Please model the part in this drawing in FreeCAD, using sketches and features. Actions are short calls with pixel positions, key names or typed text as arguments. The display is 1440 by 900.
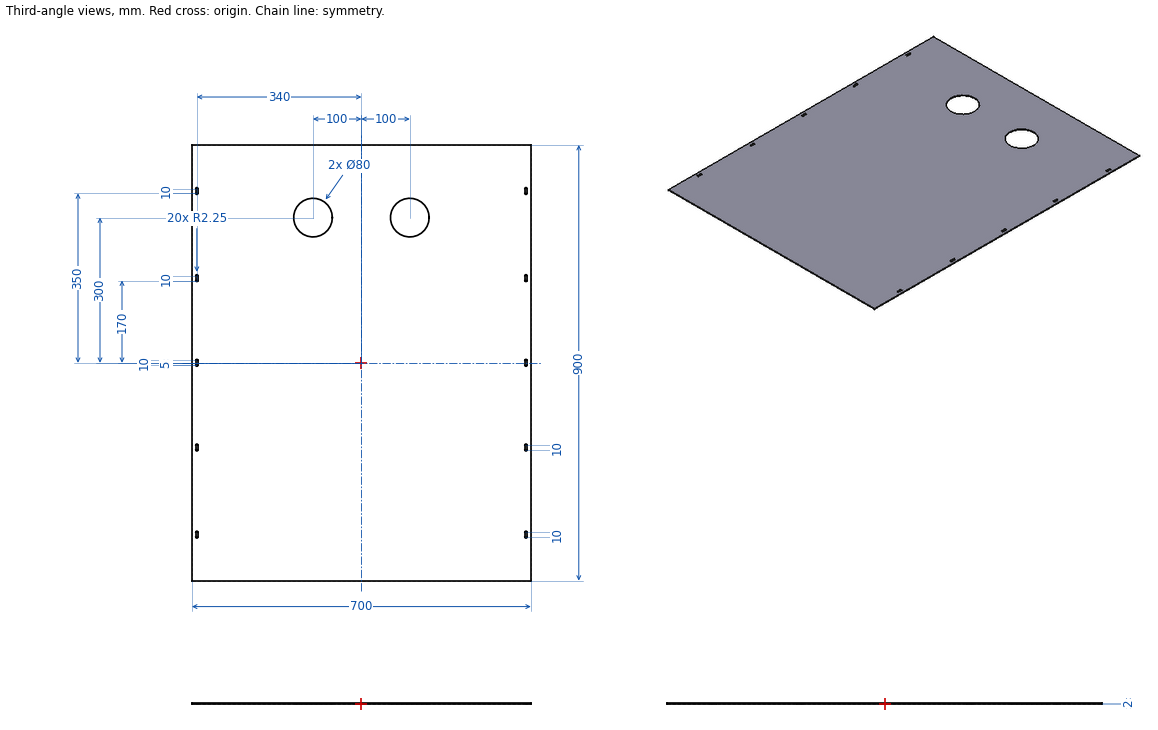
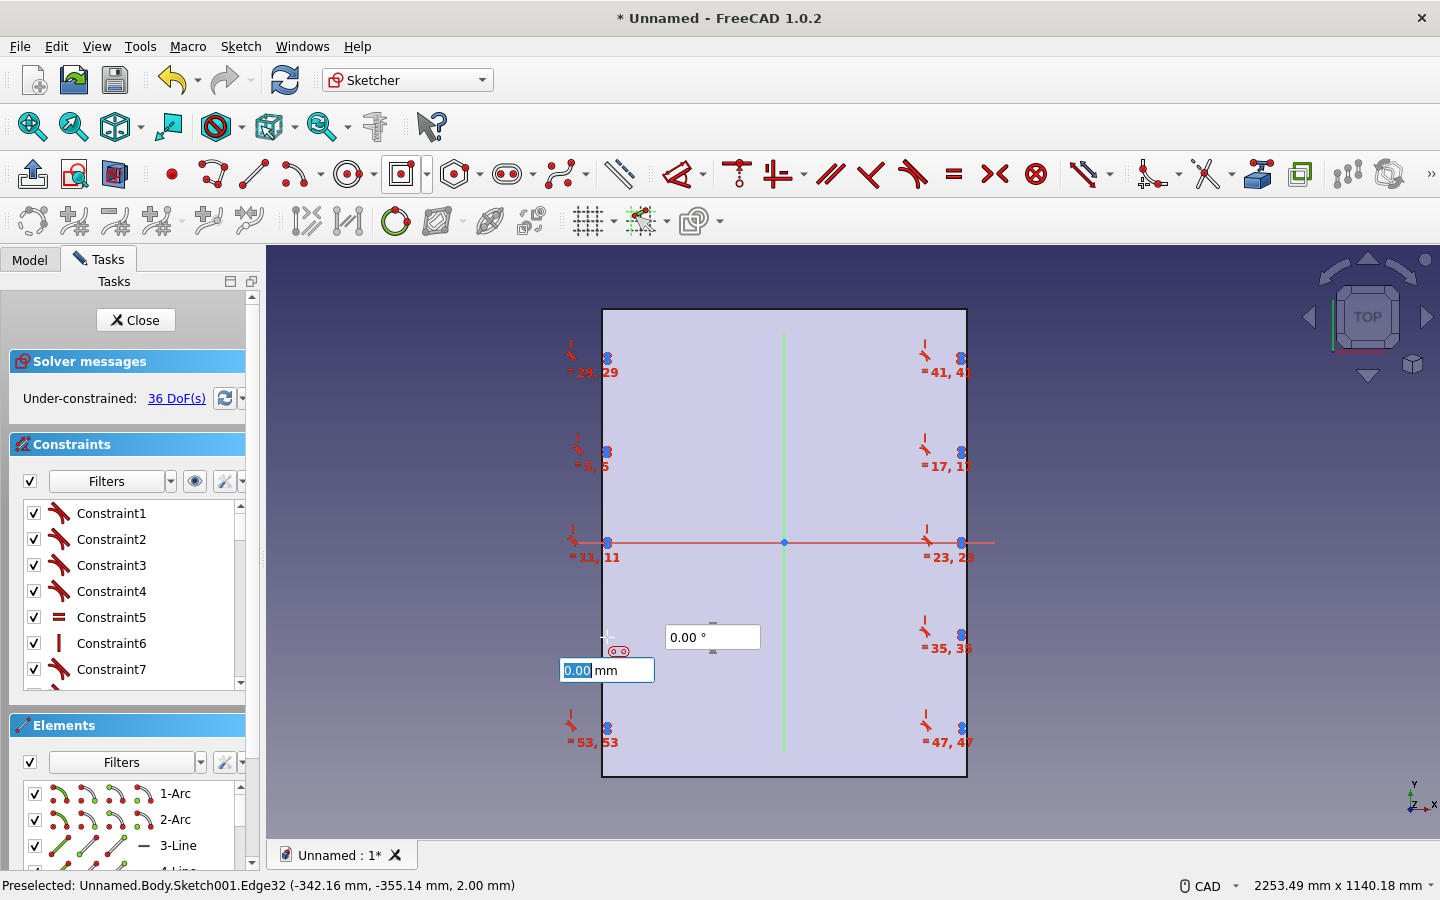
scroll(607, 632, up, 6)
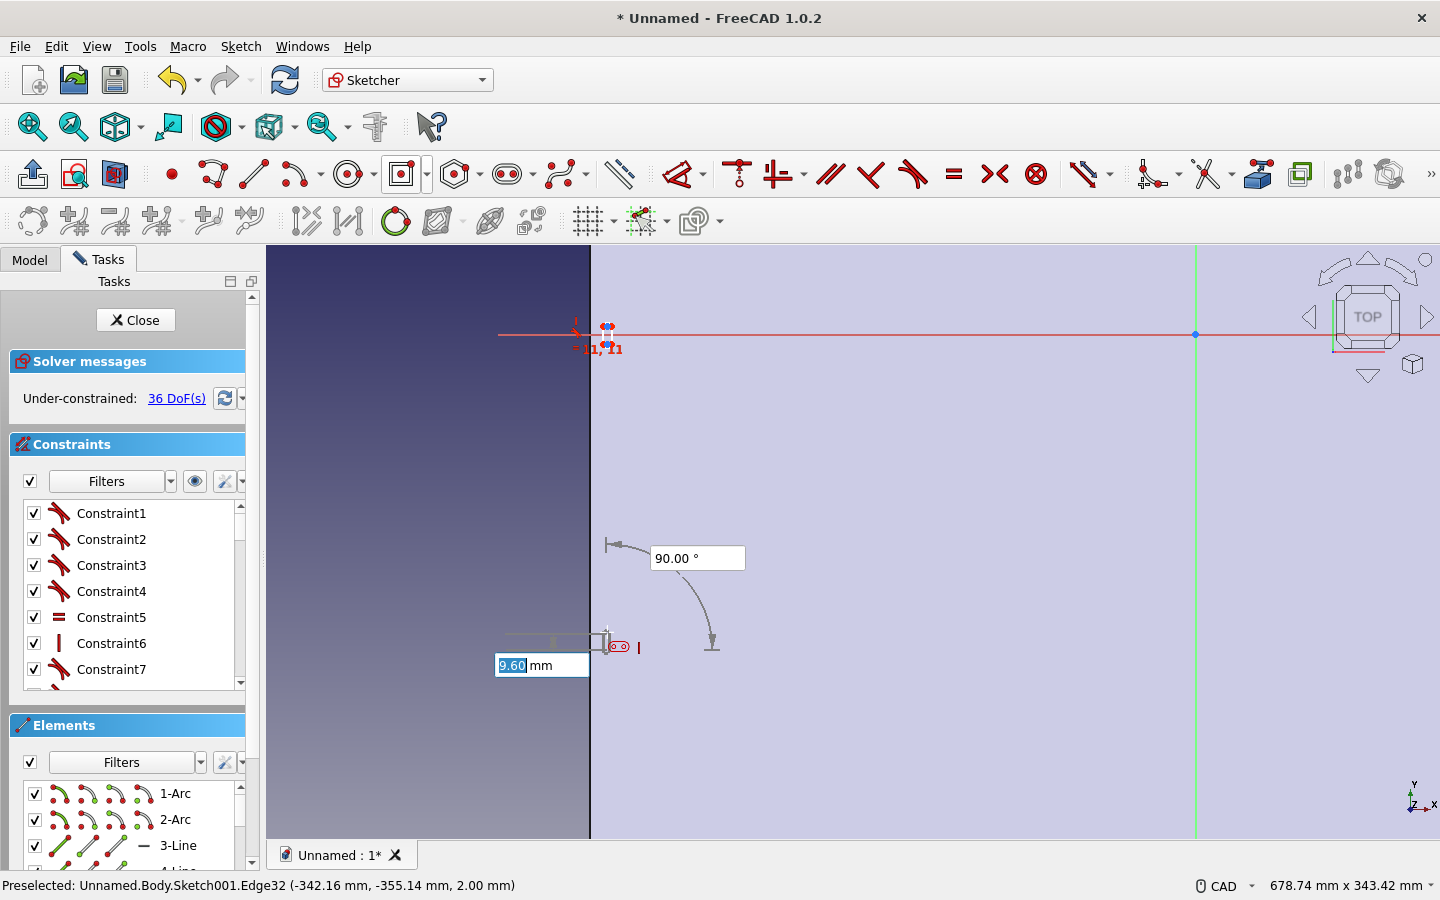
click(606, 629)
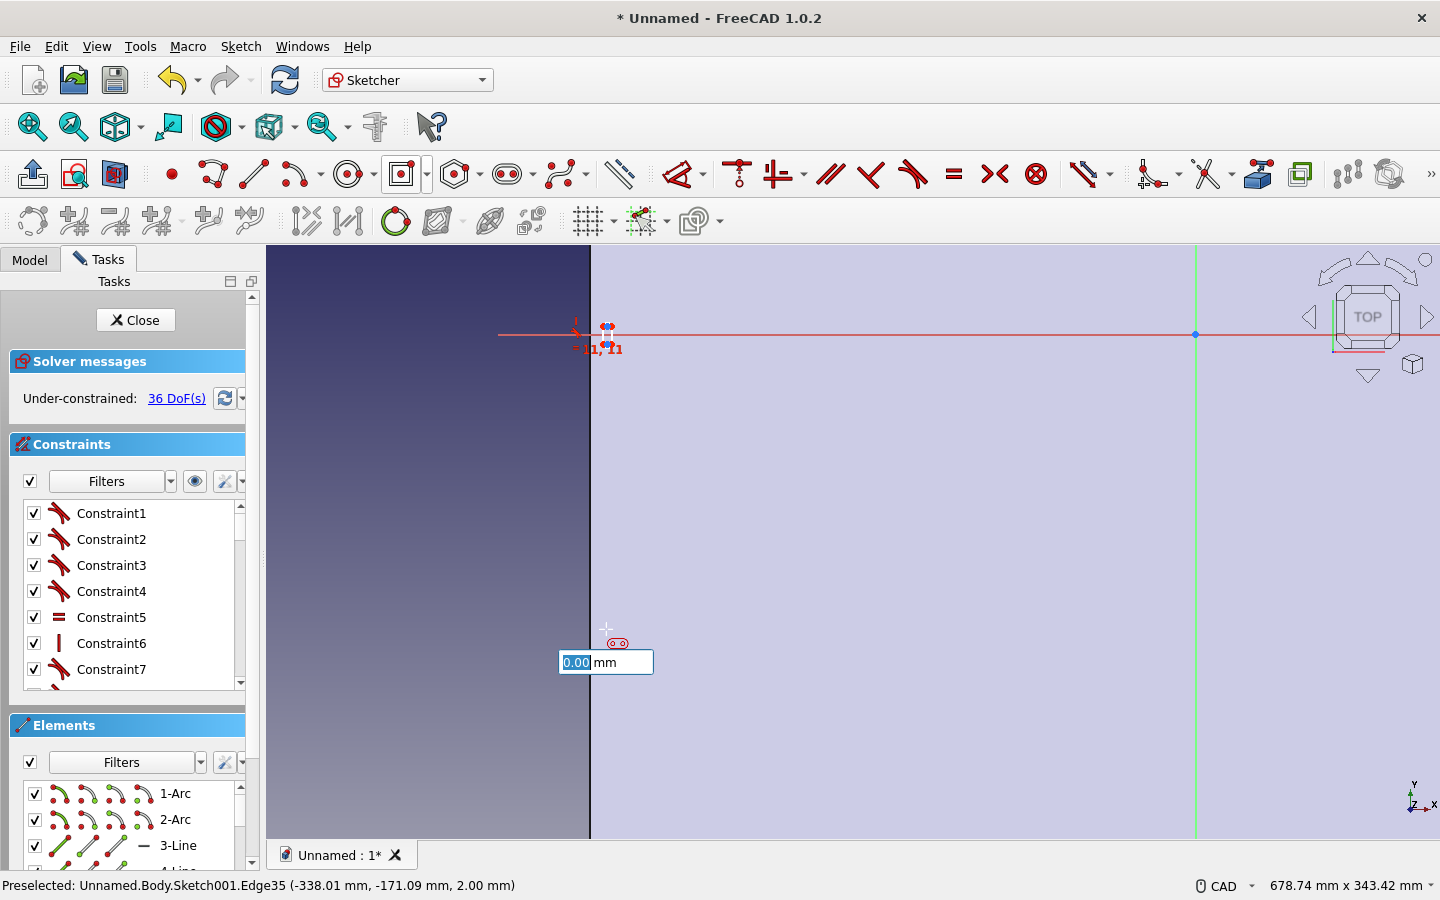
scroll(611, 638, up, 8)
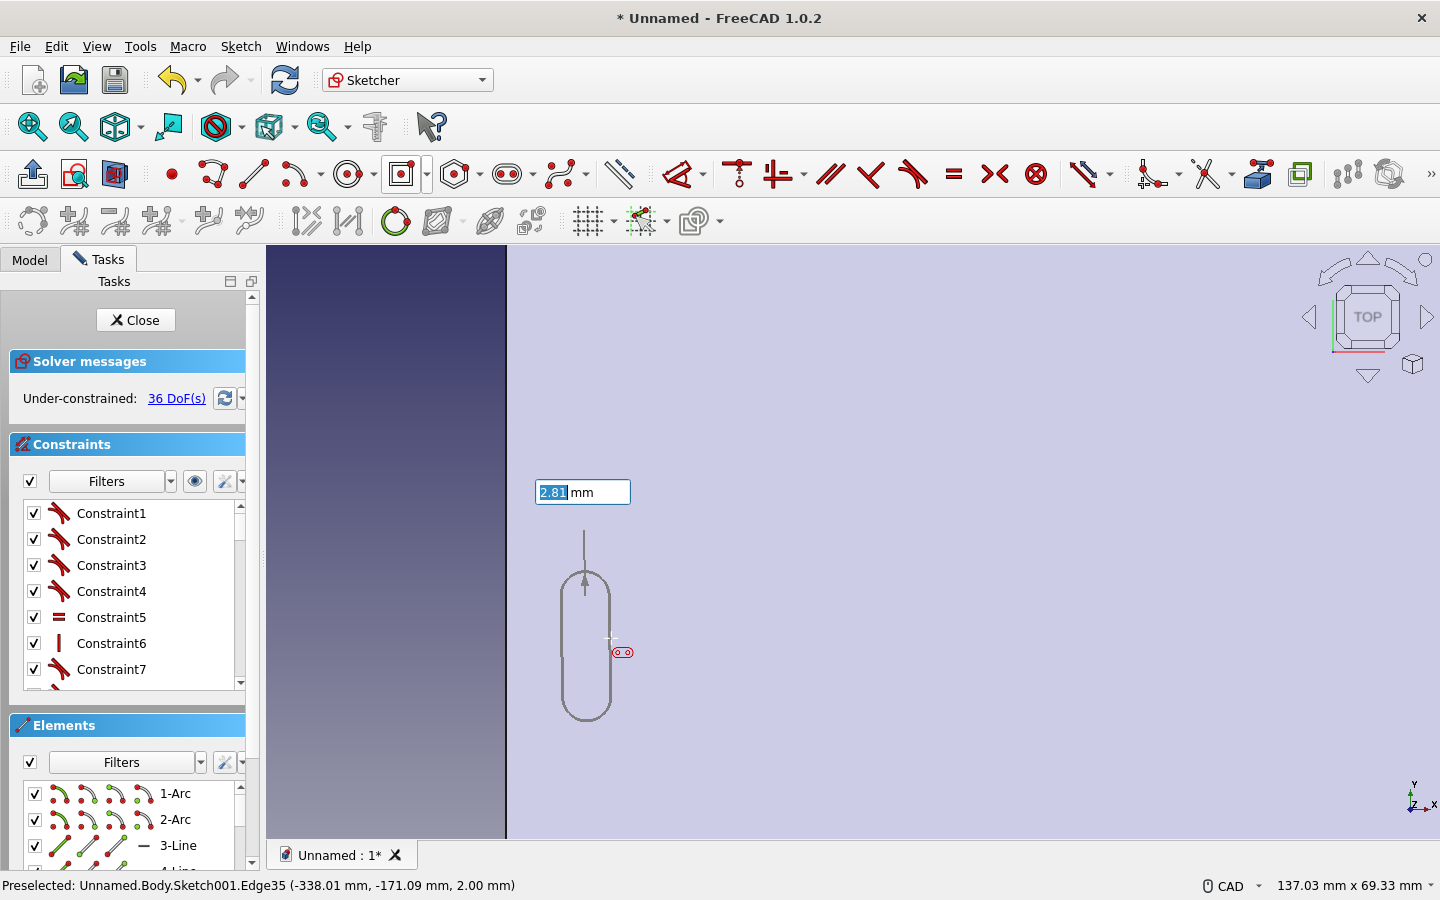
click(611, 634)
key(Escape)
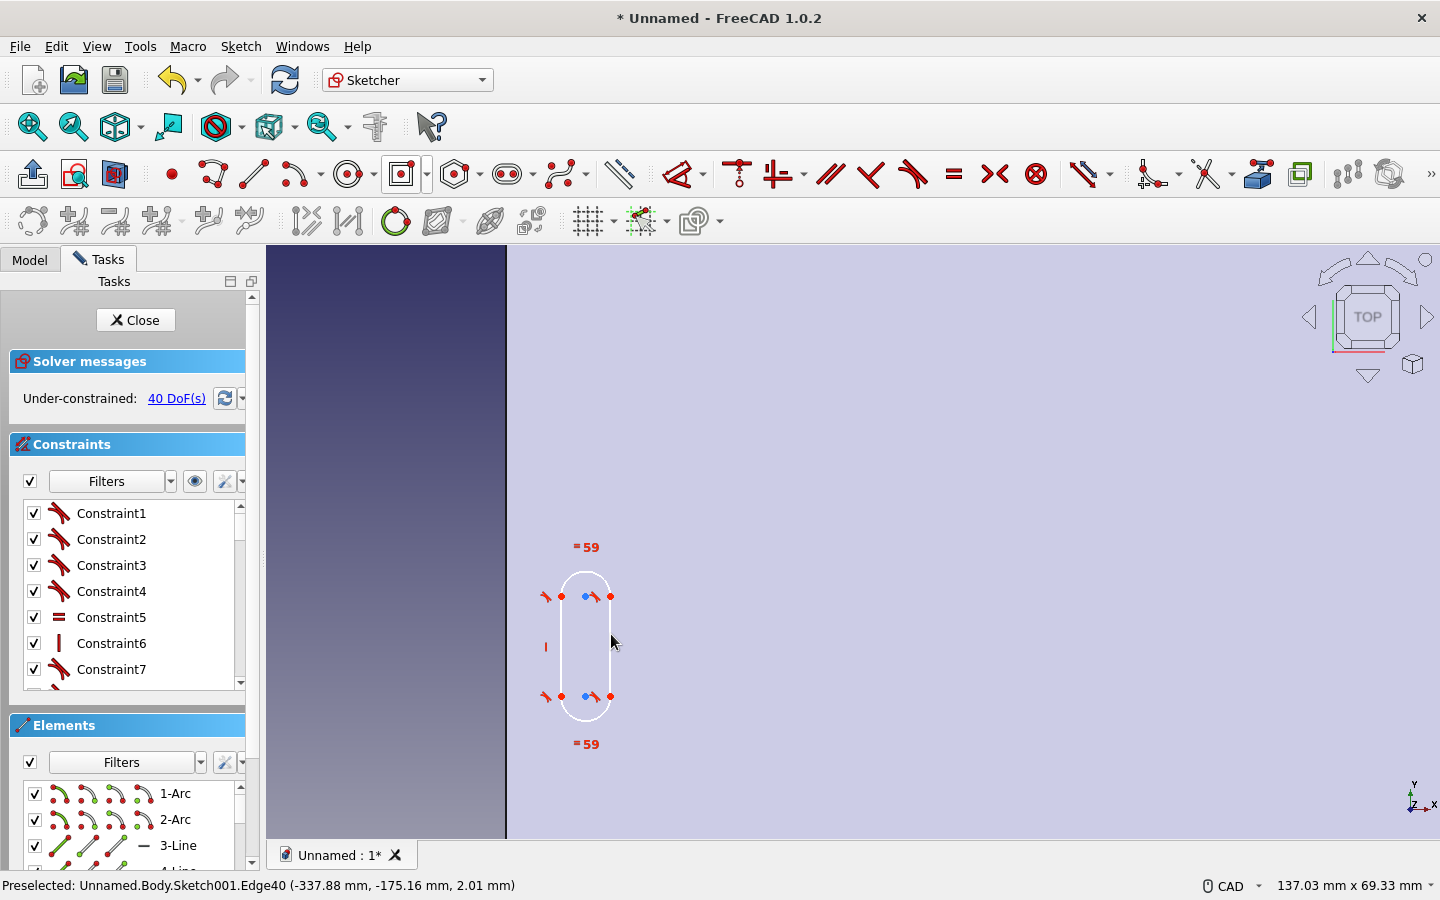
scroll(608, 633, down, 14)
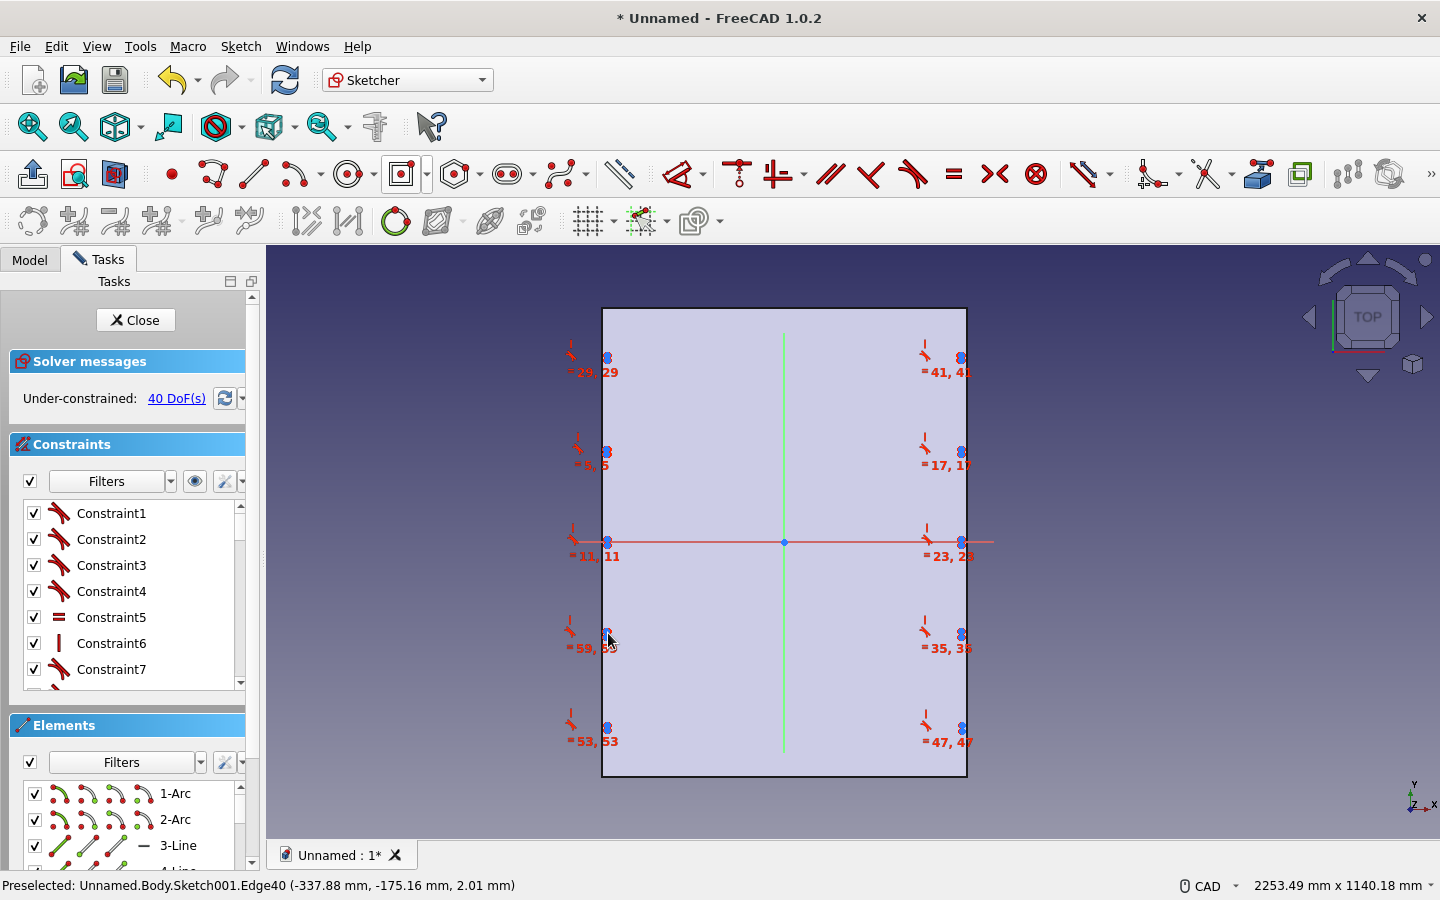
scroll(606, 456, up, 12)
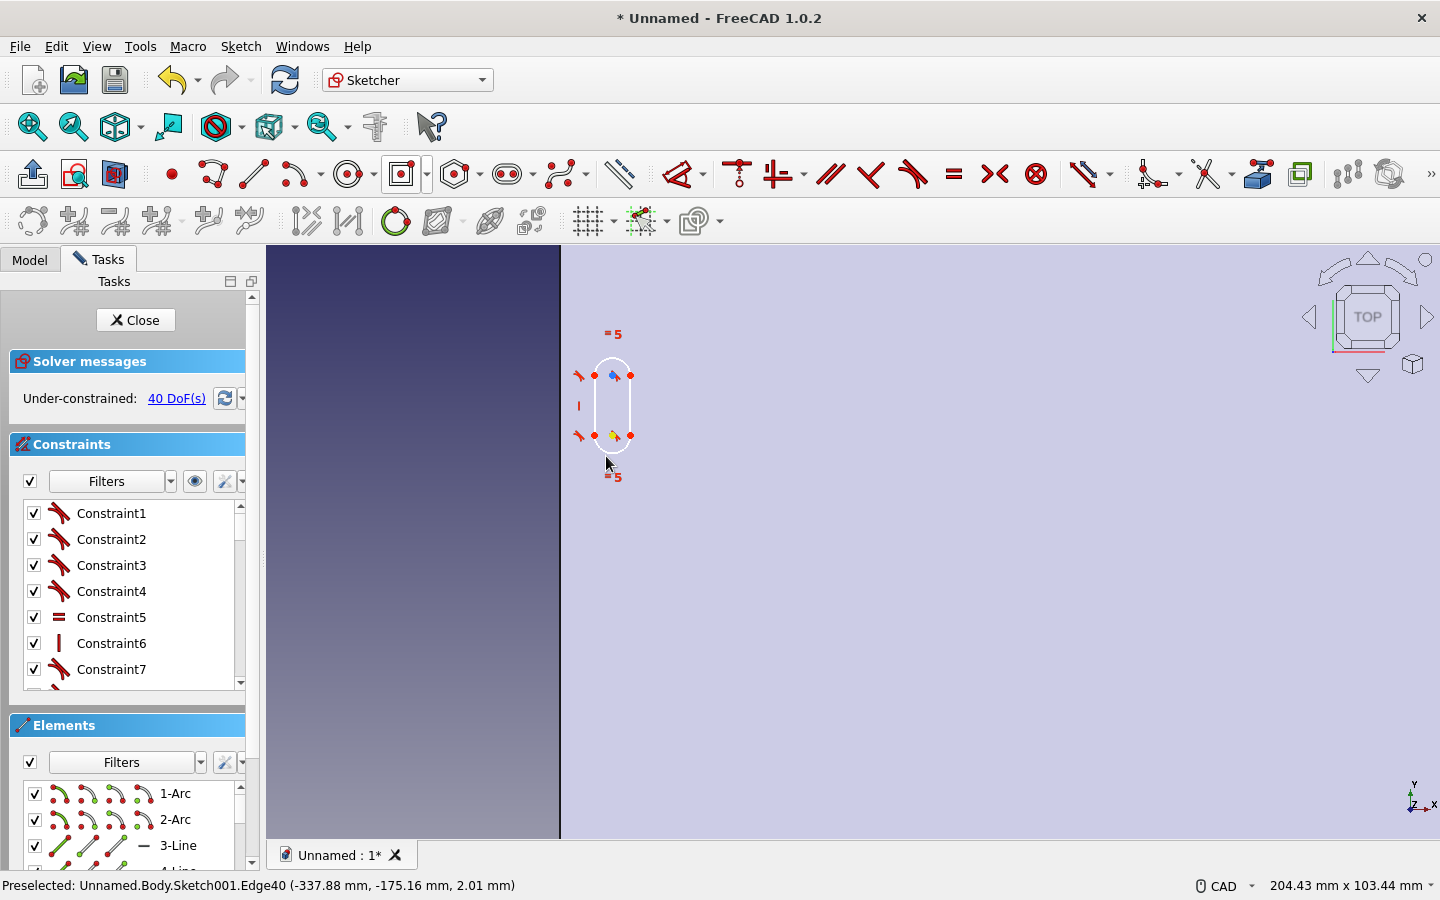
click(602, 450)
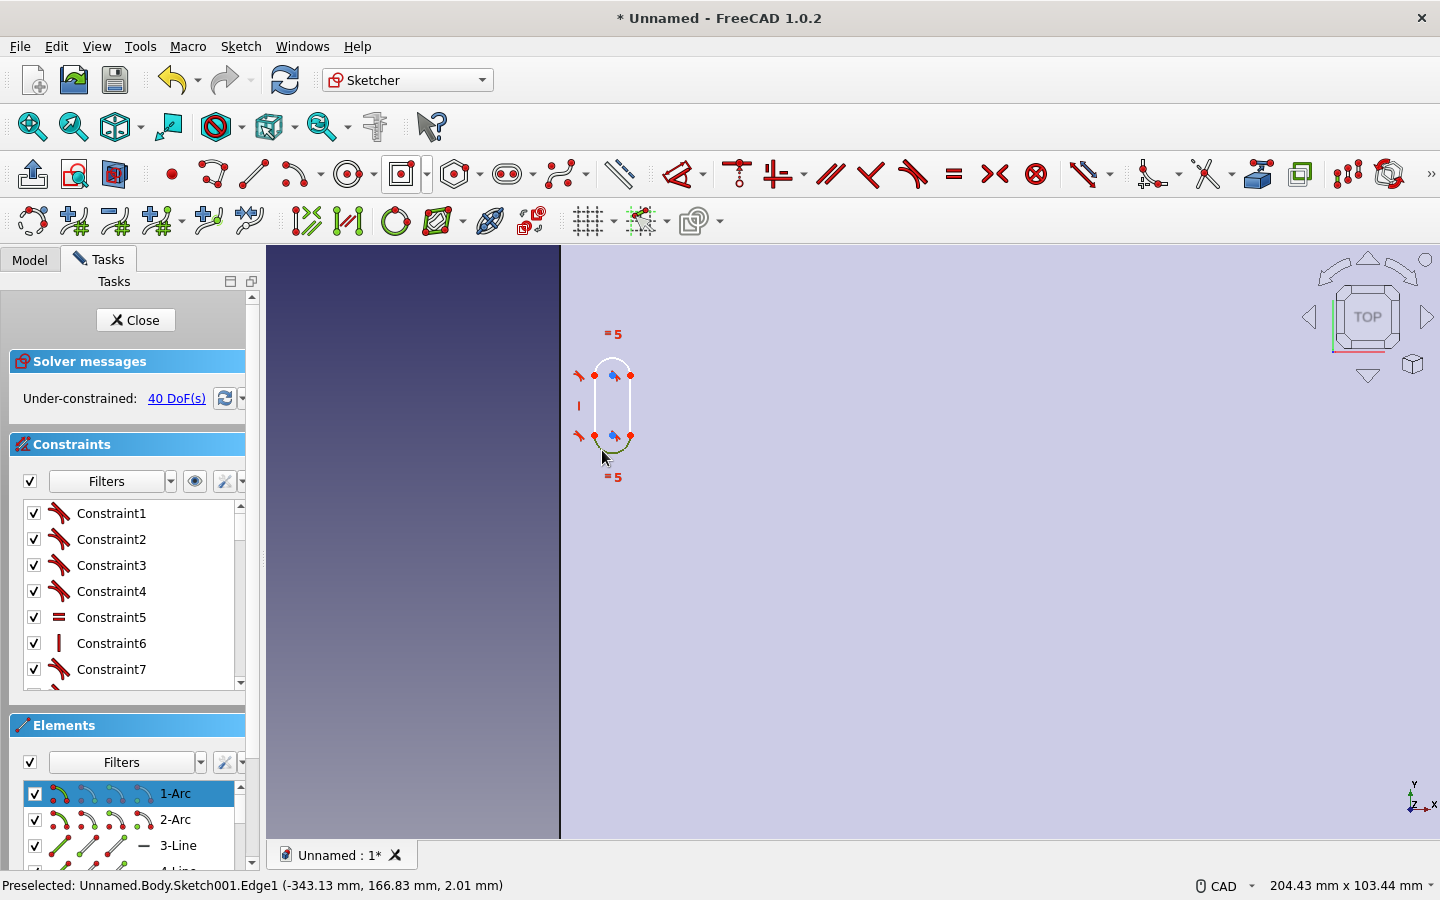
scroll(606, 456, down, 12)